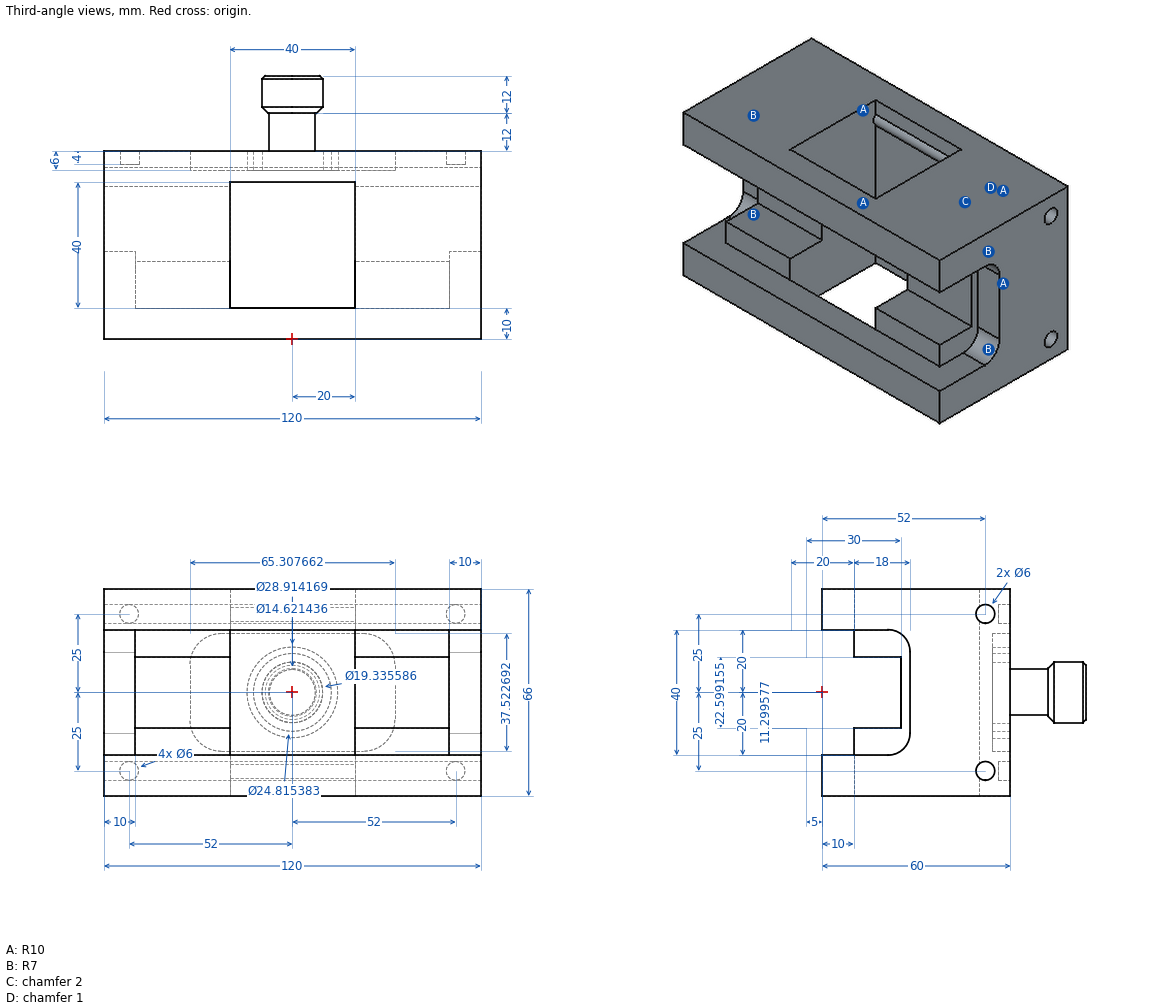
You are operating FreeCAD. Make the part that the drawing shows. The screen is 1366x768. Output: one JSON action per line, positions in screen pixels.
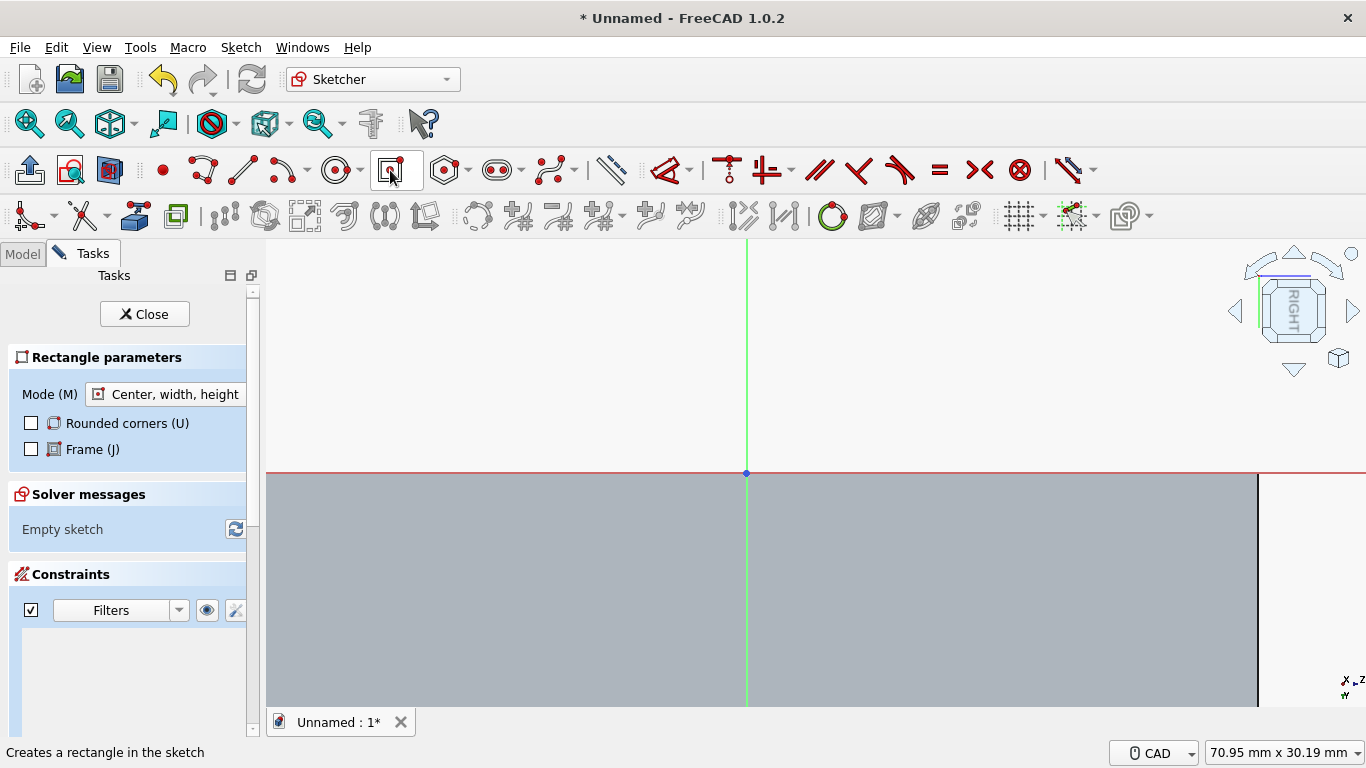
{"action": "left_click", "coordinate": [747, 473]}
{"action": "mouse_move", "coordinate": [1057, 318]}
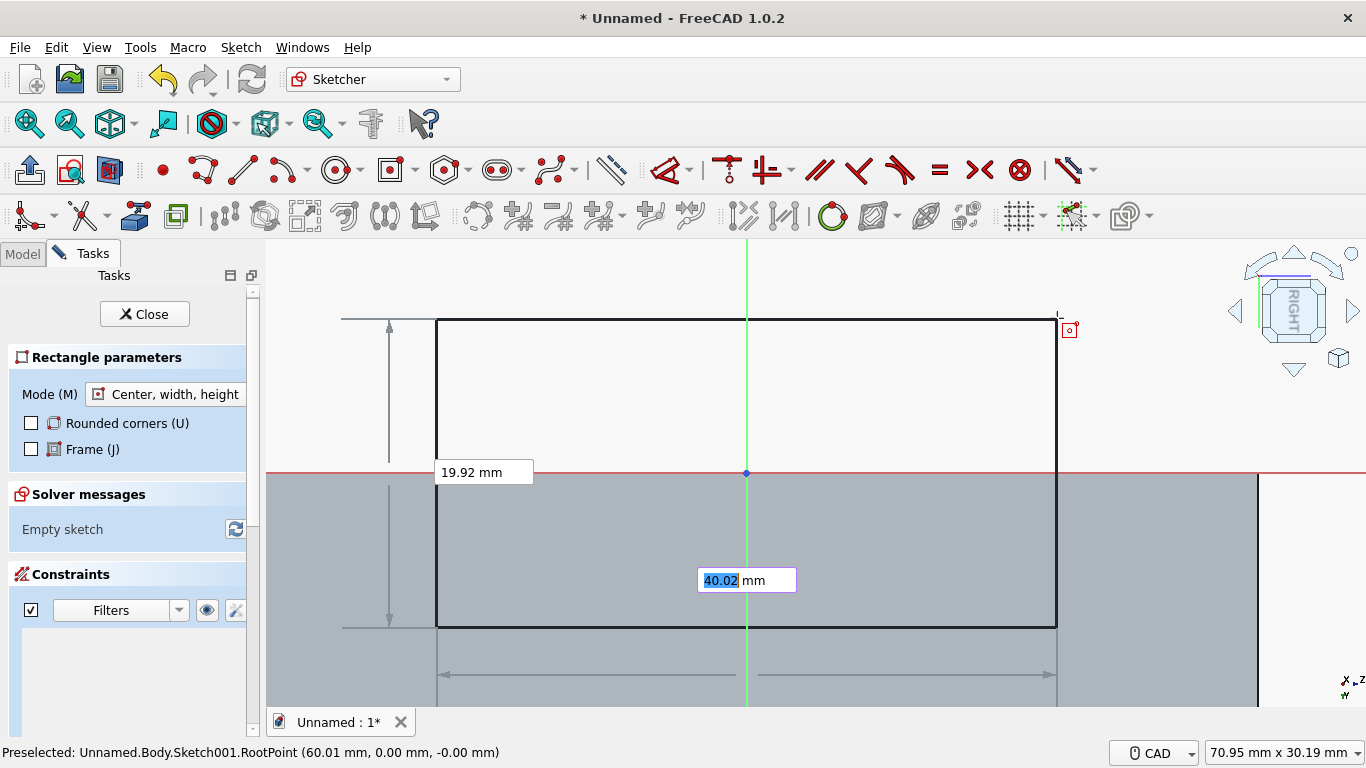
{"action": "type", "text": "40"}
{"action": "key", "text": "Tab"}
{"action": "type", "text": "20"}
{"action": "key", "text": "Return"}
{"action": "key", "text": "Escape"}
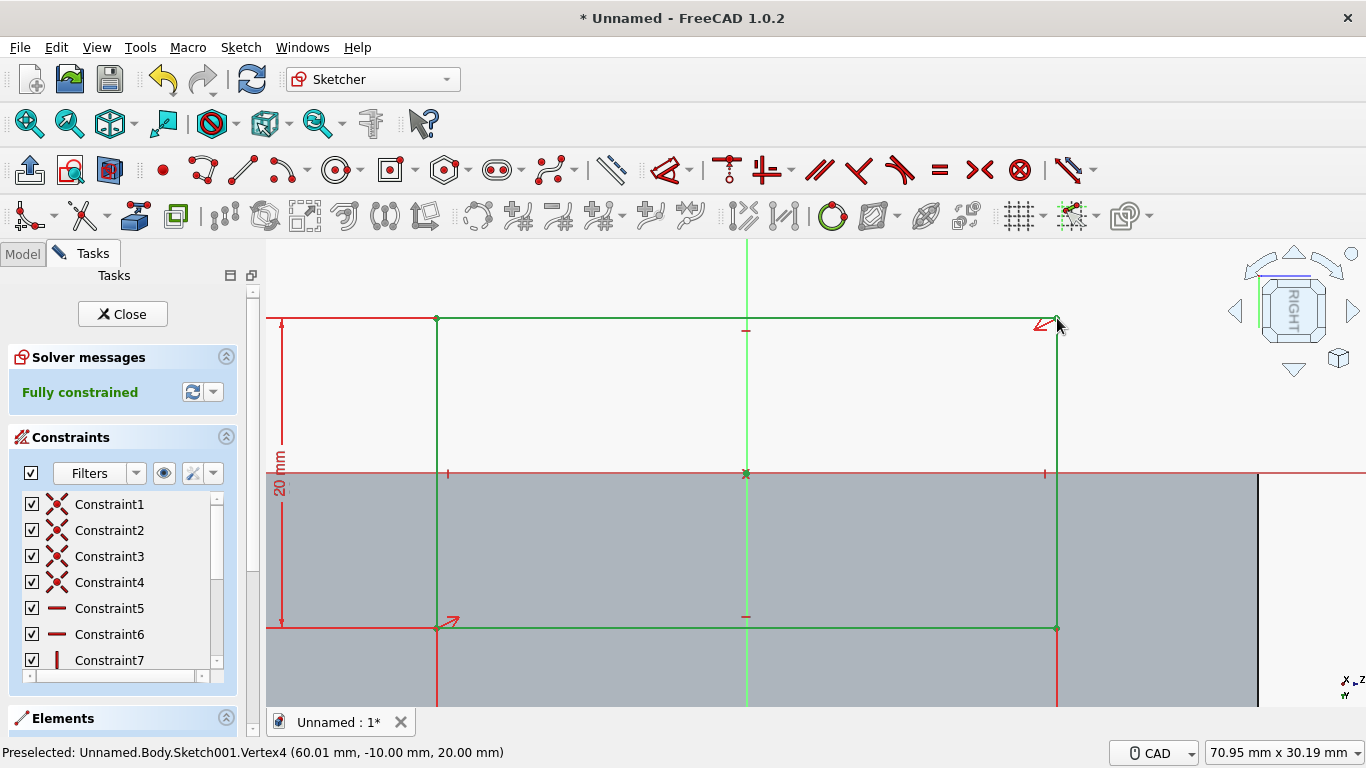
{"action": "left_click", "coordinate": [123, 314]}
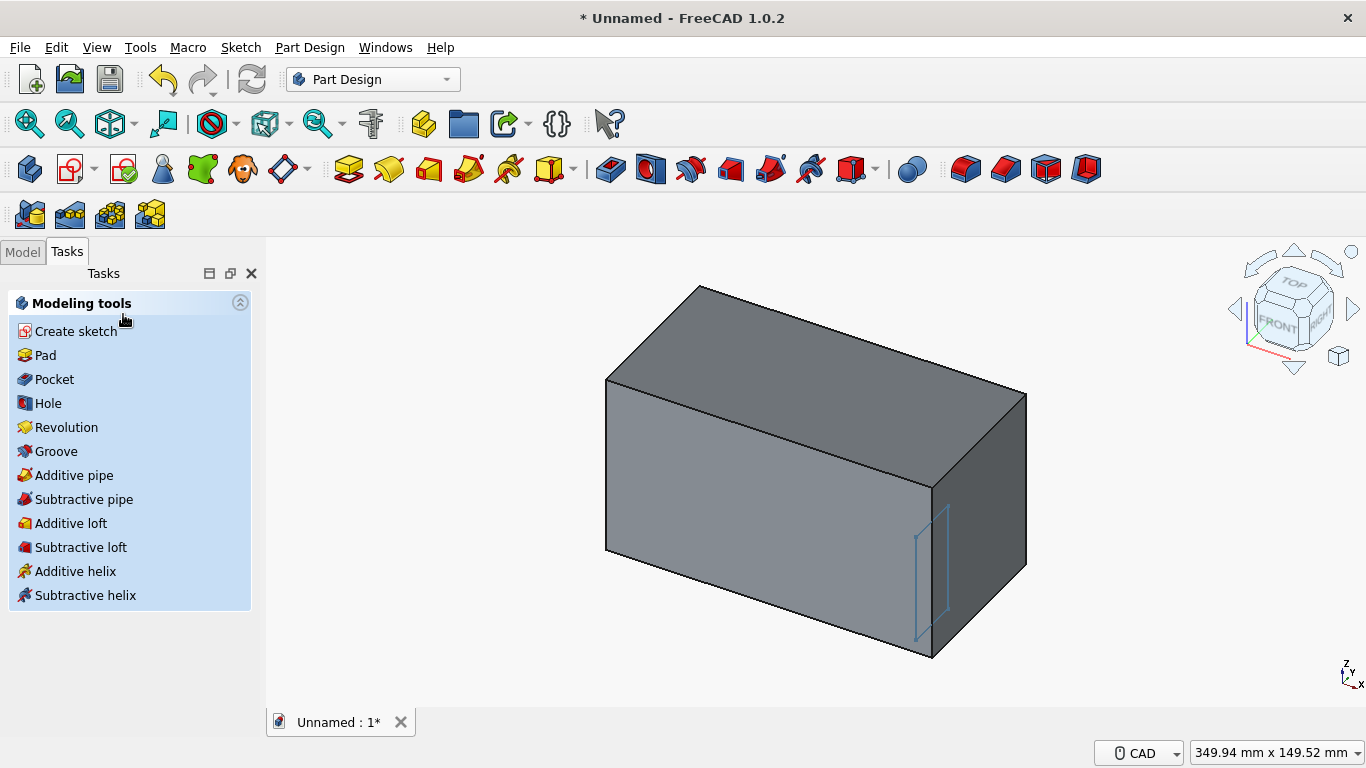
{"action": "left_click", "coordinate": [612, 170]}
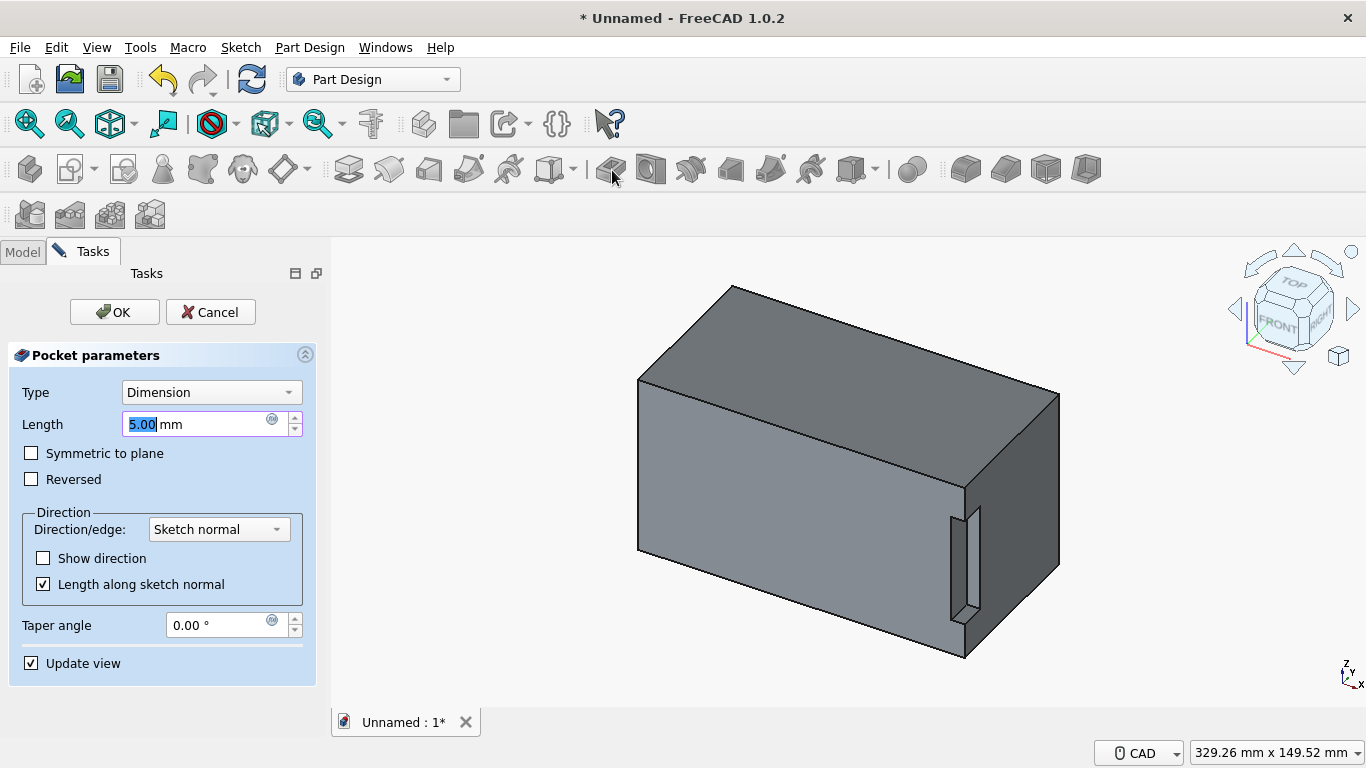
{"action": "type", "text": "120"}
{"action": "key", "text": "Tab"}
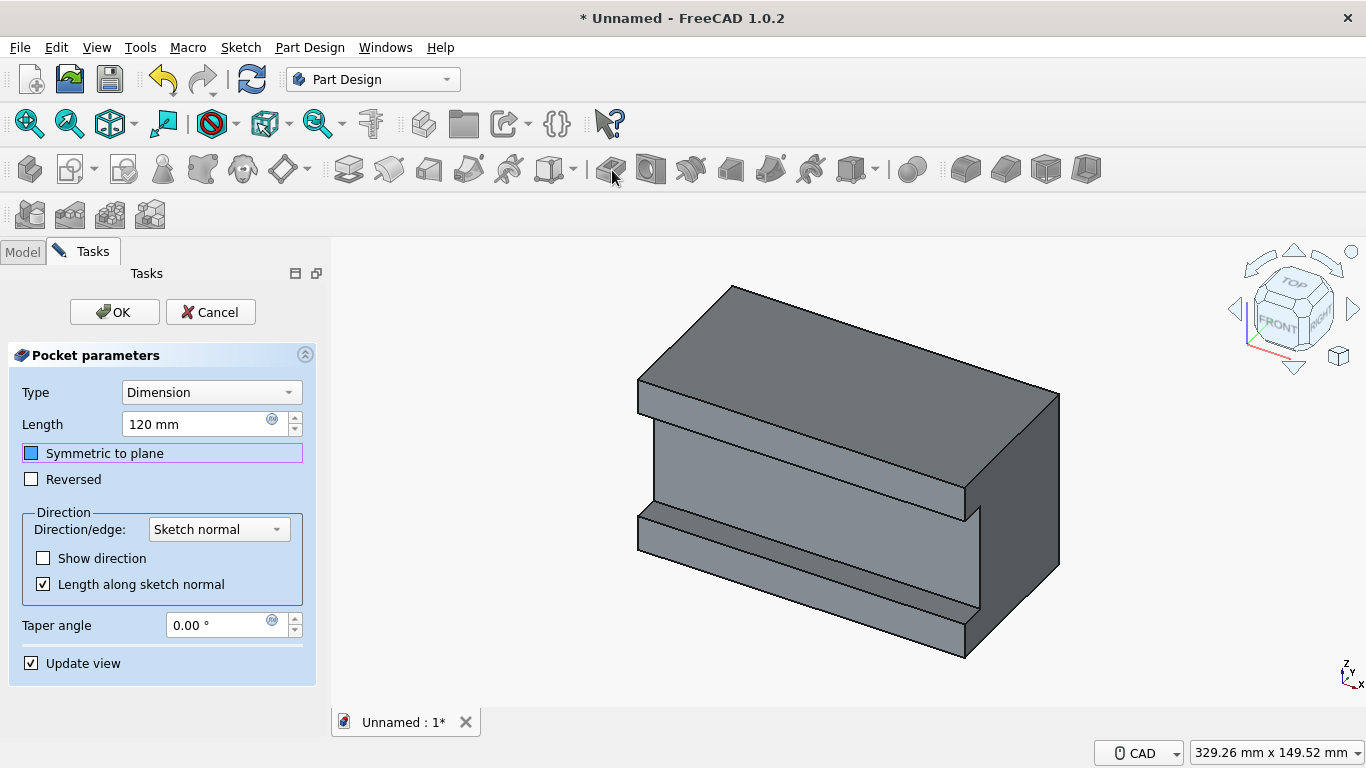
{"action": "left_click", "coordinate": [115, 312]}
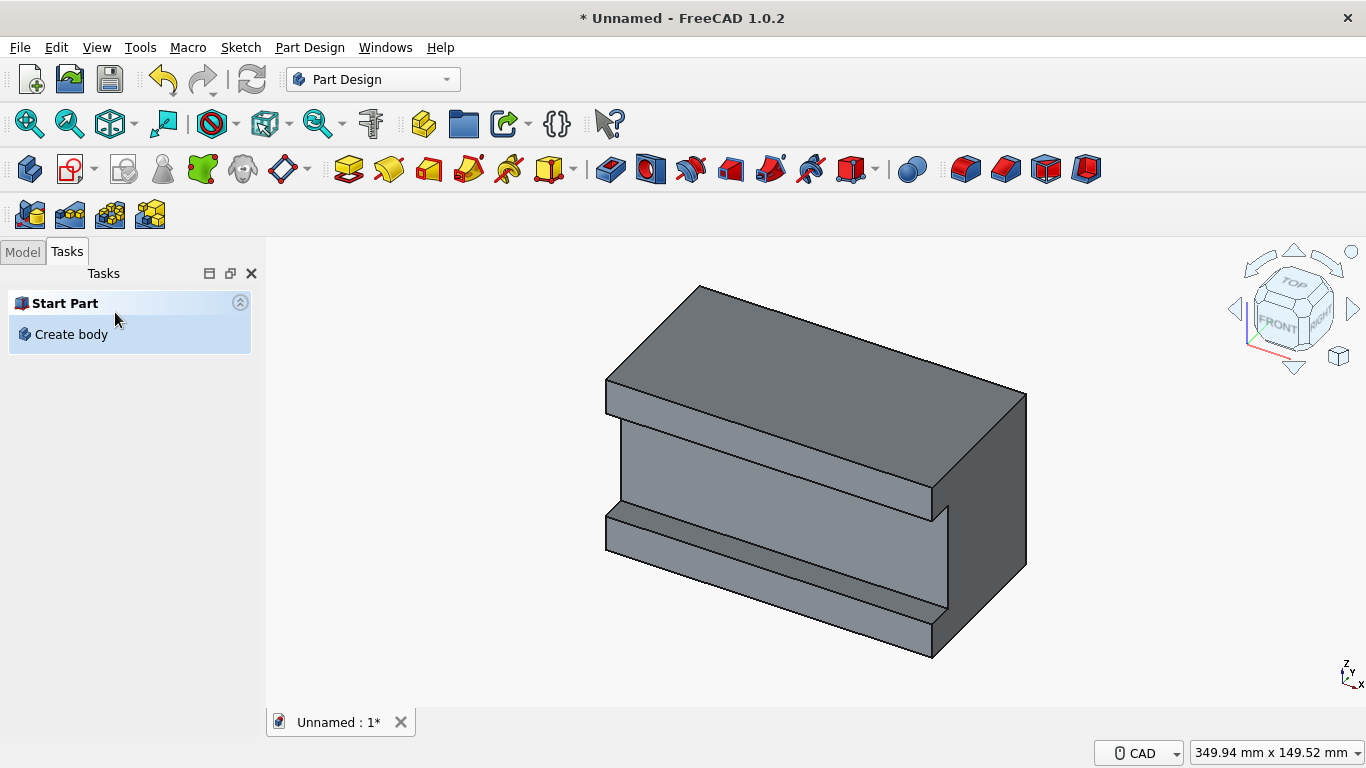
{"action": "left_click", "coordinate": [863, 401]}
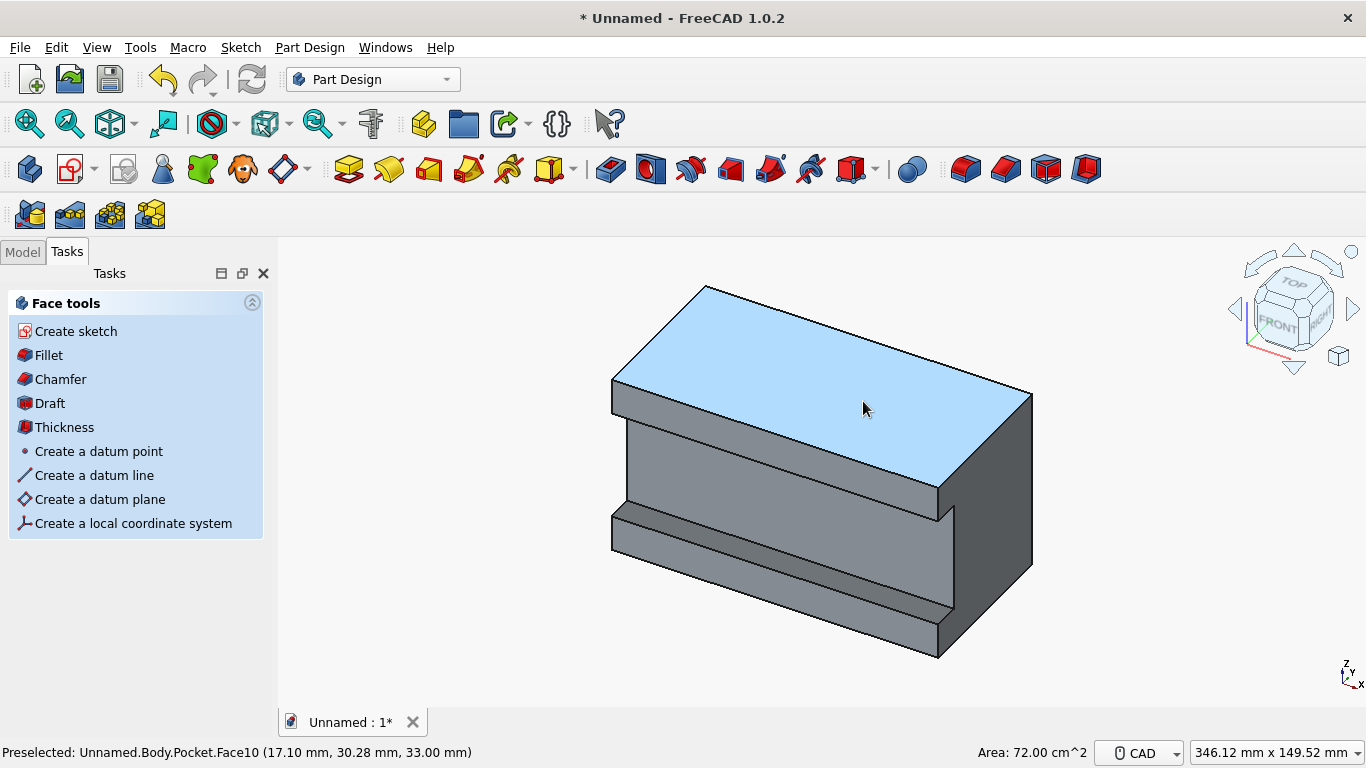
{"action": "left_click", "coordinate": [70, 170]}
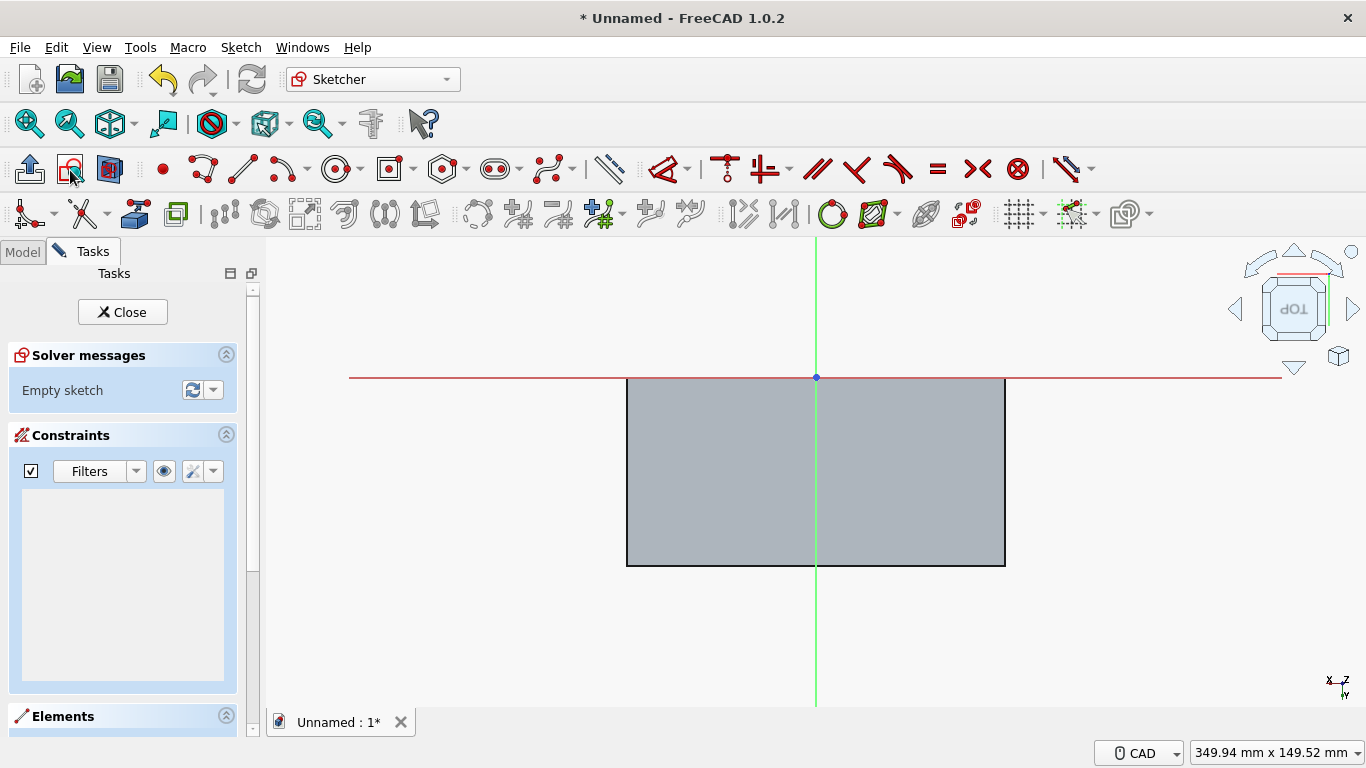
{"action": "scroll", "coordinate": [899, 437], "scroll_direction": "up", "scroll_amount": 3}